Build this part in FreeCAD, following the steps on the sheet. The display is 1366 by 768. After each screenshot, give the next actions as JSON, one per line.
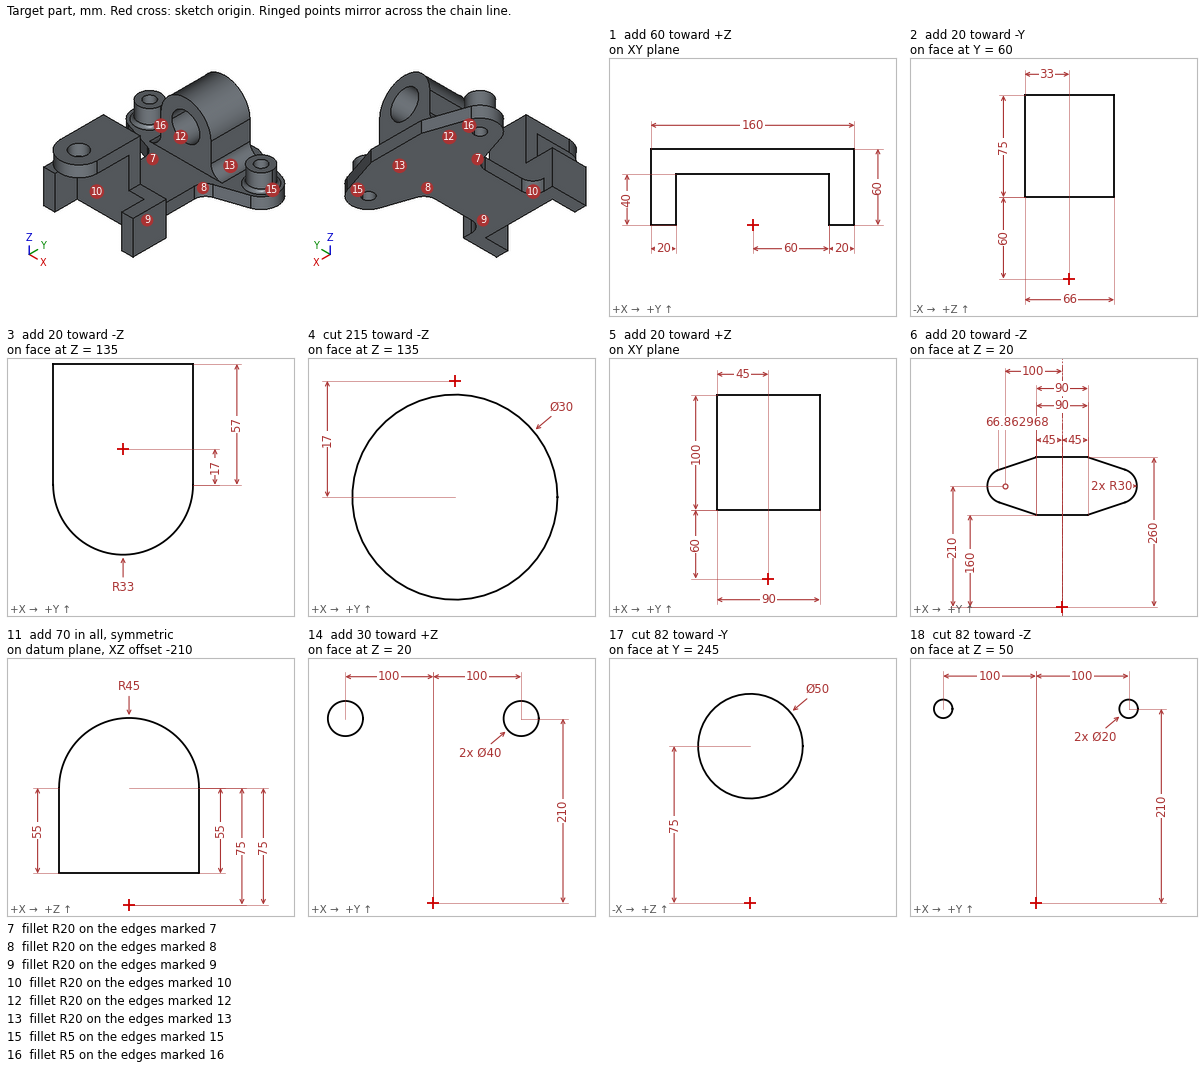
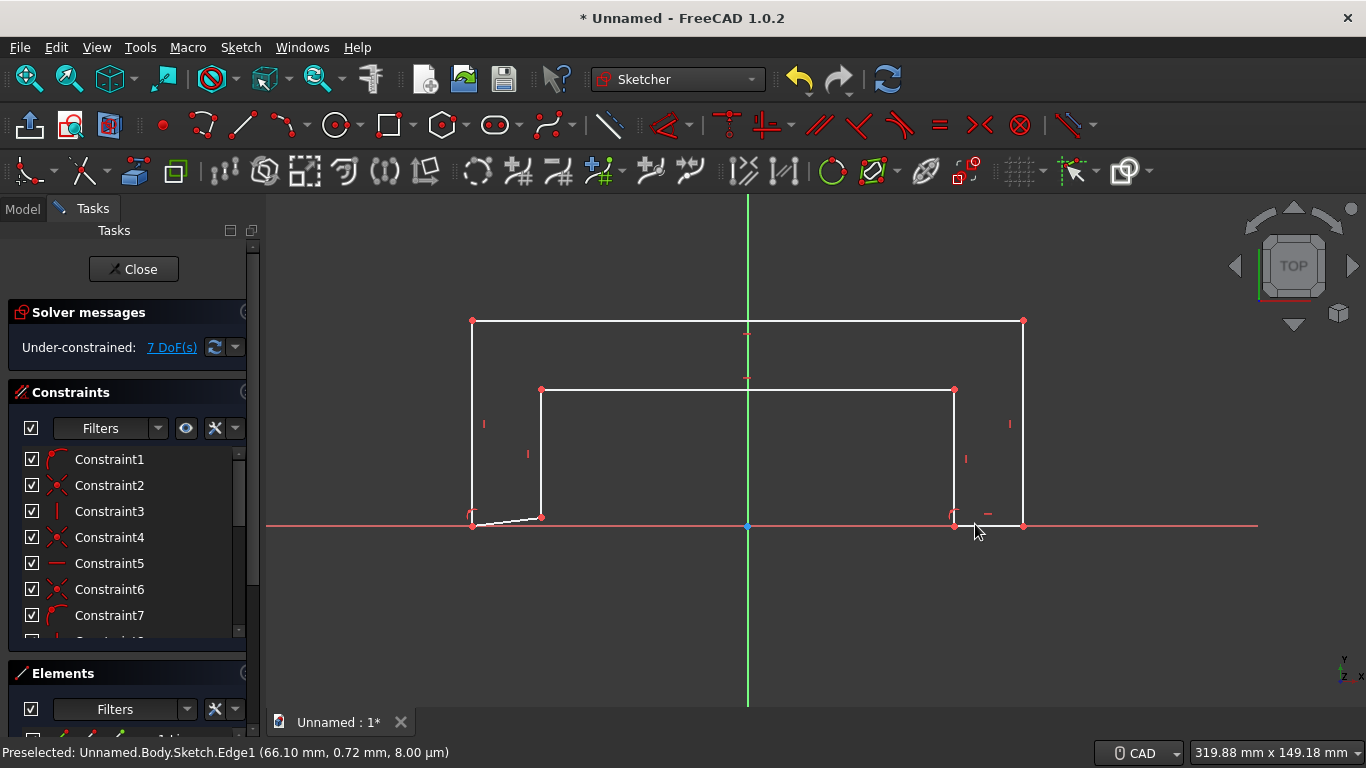
{"action": "left_click", "coordinate": [493, 524]}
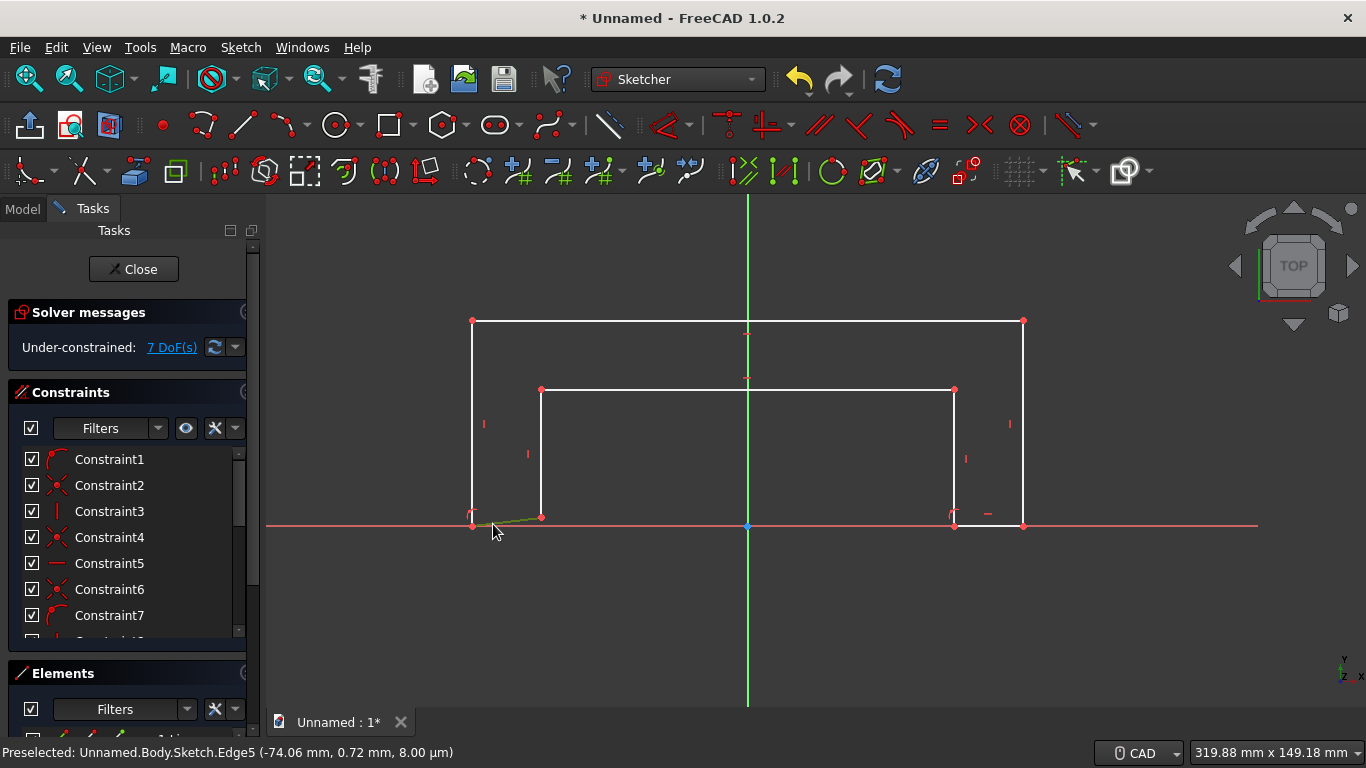
{"action": "left_click", "coordinate": [794, 126]}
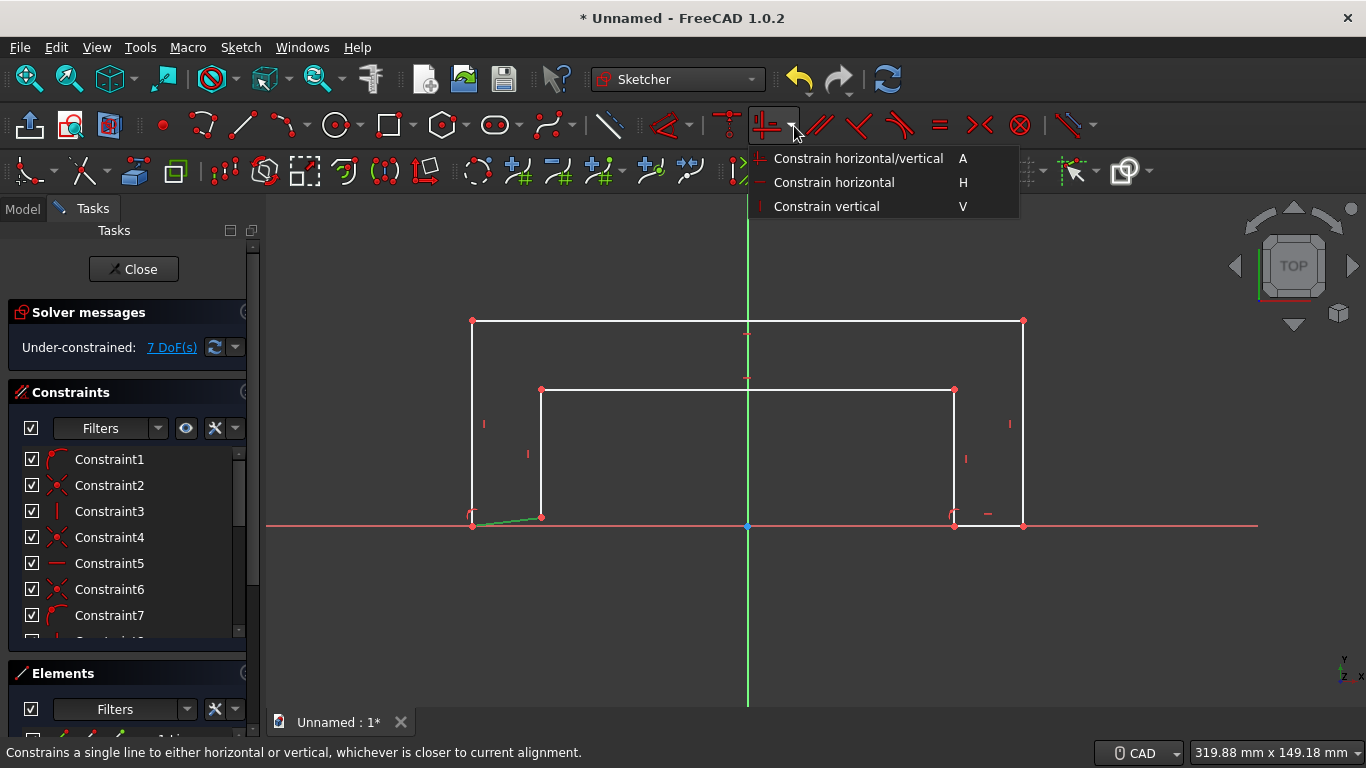
{"action": "left_click", "coordinate": [884, 182]}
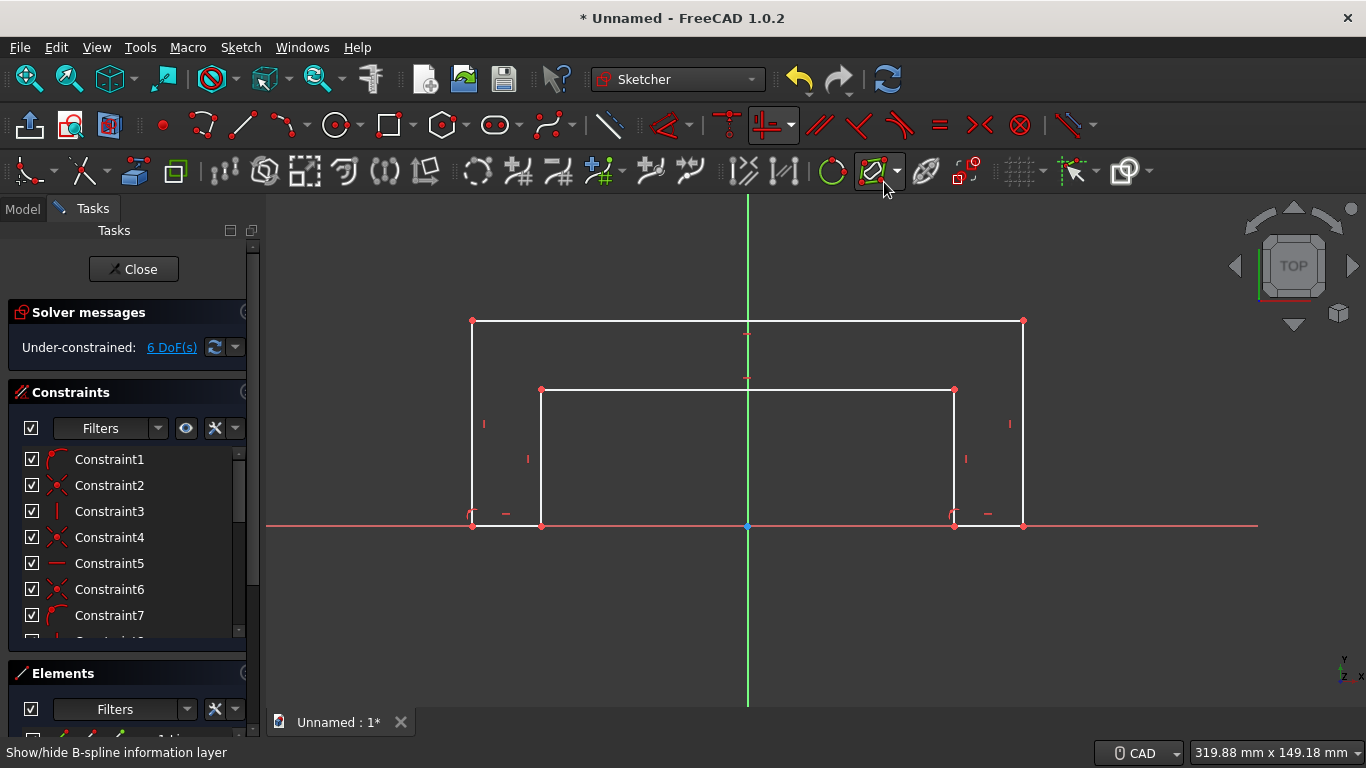
{"action": "left_click", "coordinate": [664, 126]}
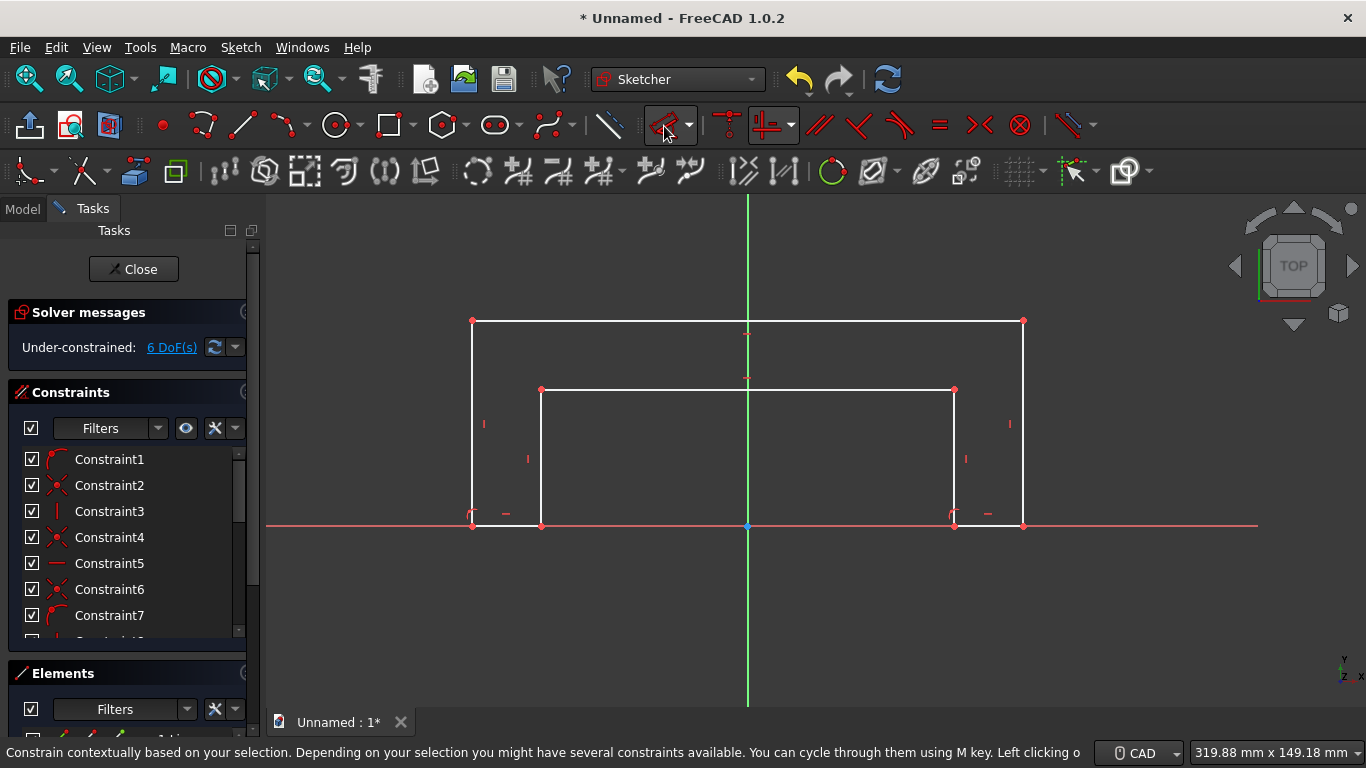
{"action": "left_click", "coordinate": [975, 526]}
{"action": "left_click", "coordinate": [989, 560]}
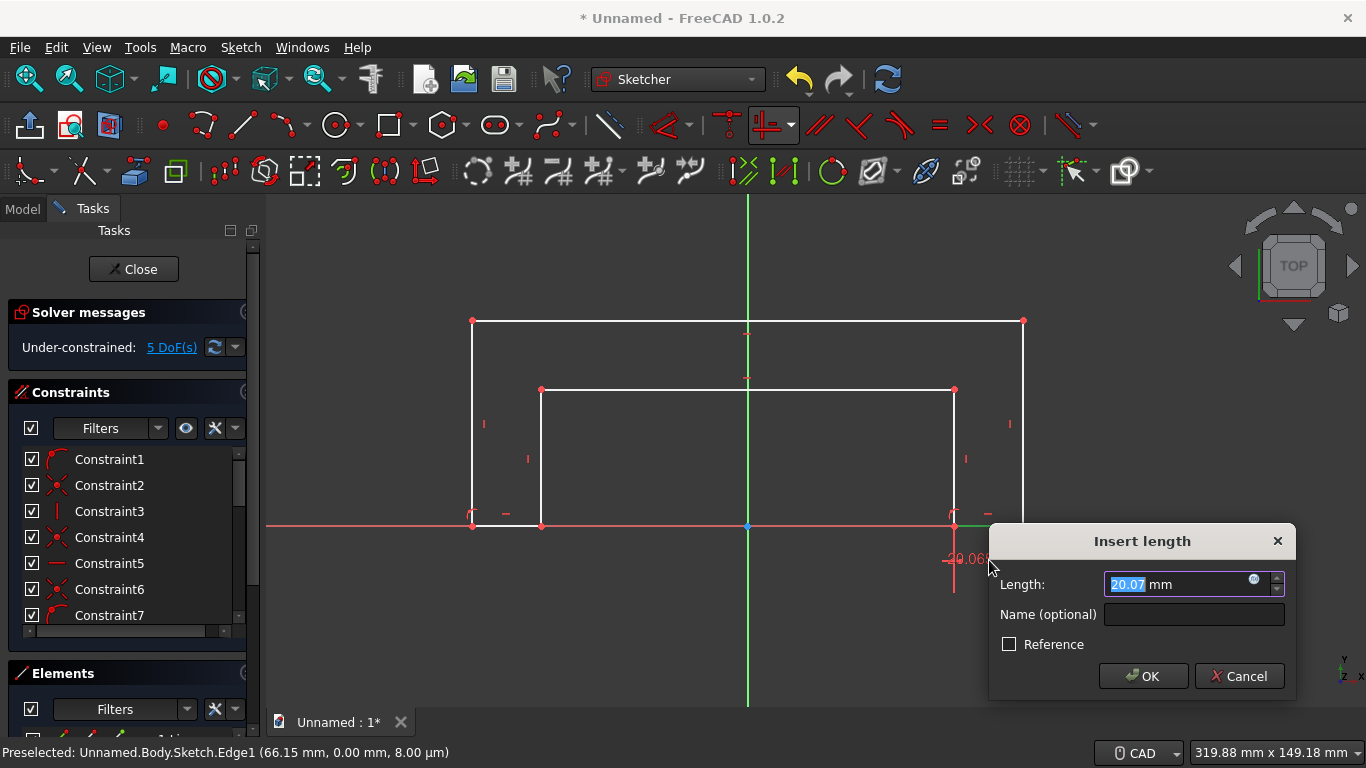
{"action": "type", "text": "20"}
{"action": "key", "text": "Return"}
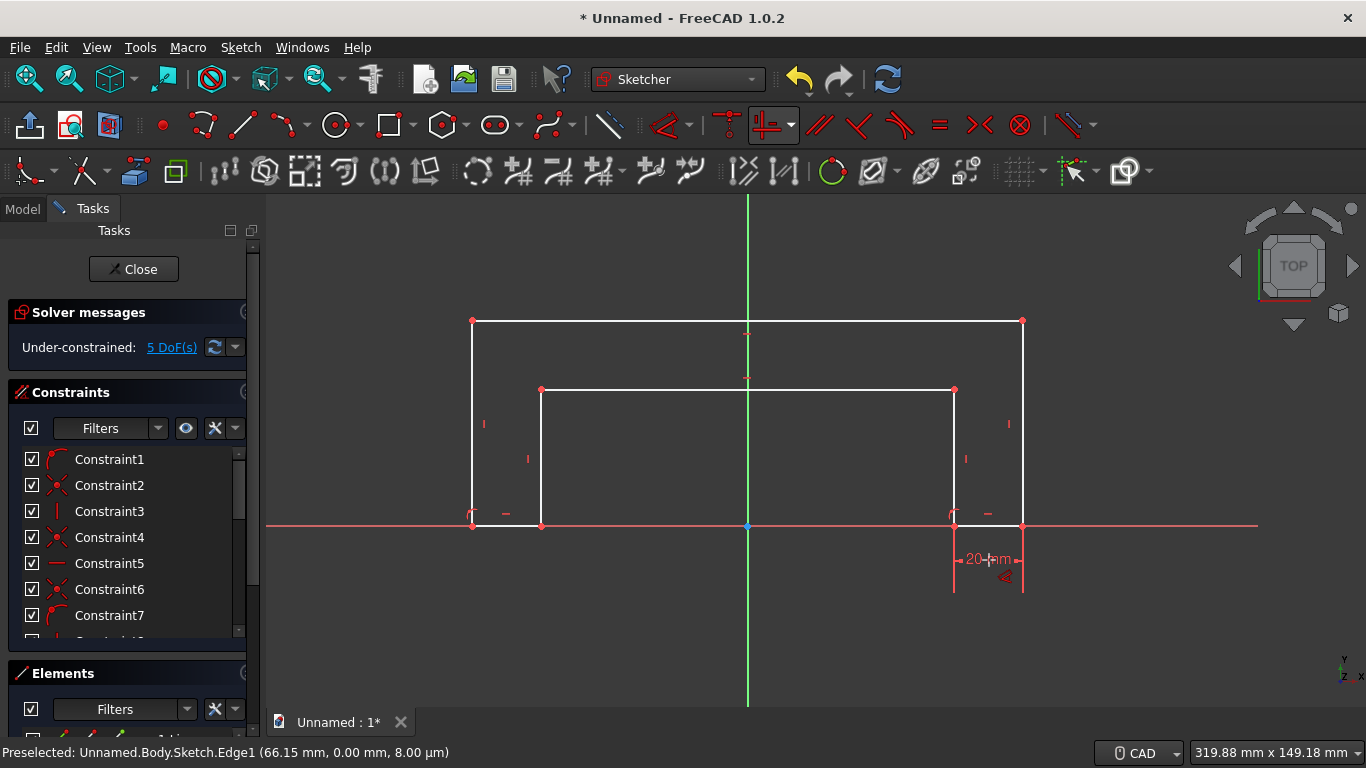
{"action": "left_click", "coordinate": [1023, 465]}
{"action": "left_click", "coordinate": [1057, 424]}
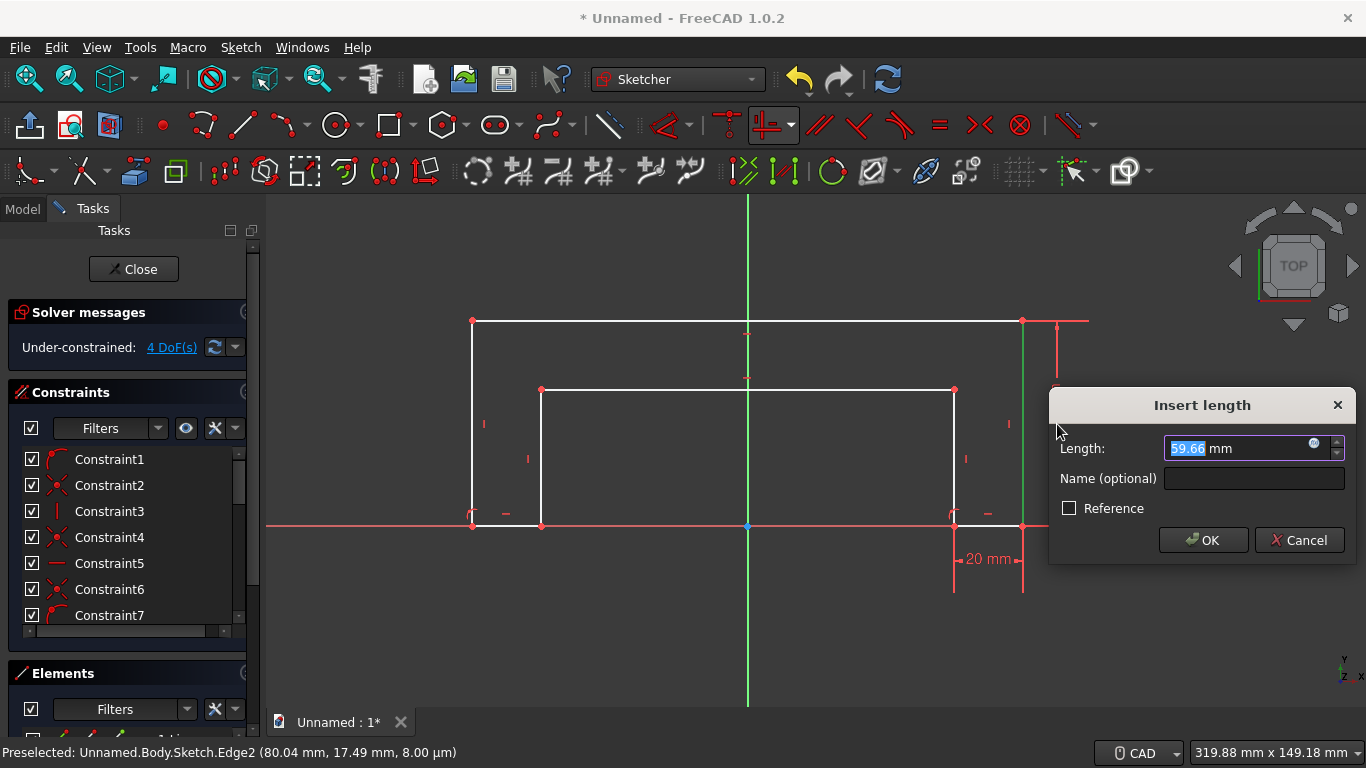
{"action": "type", "text": "60"}
{"action": "key", "text": "Return"}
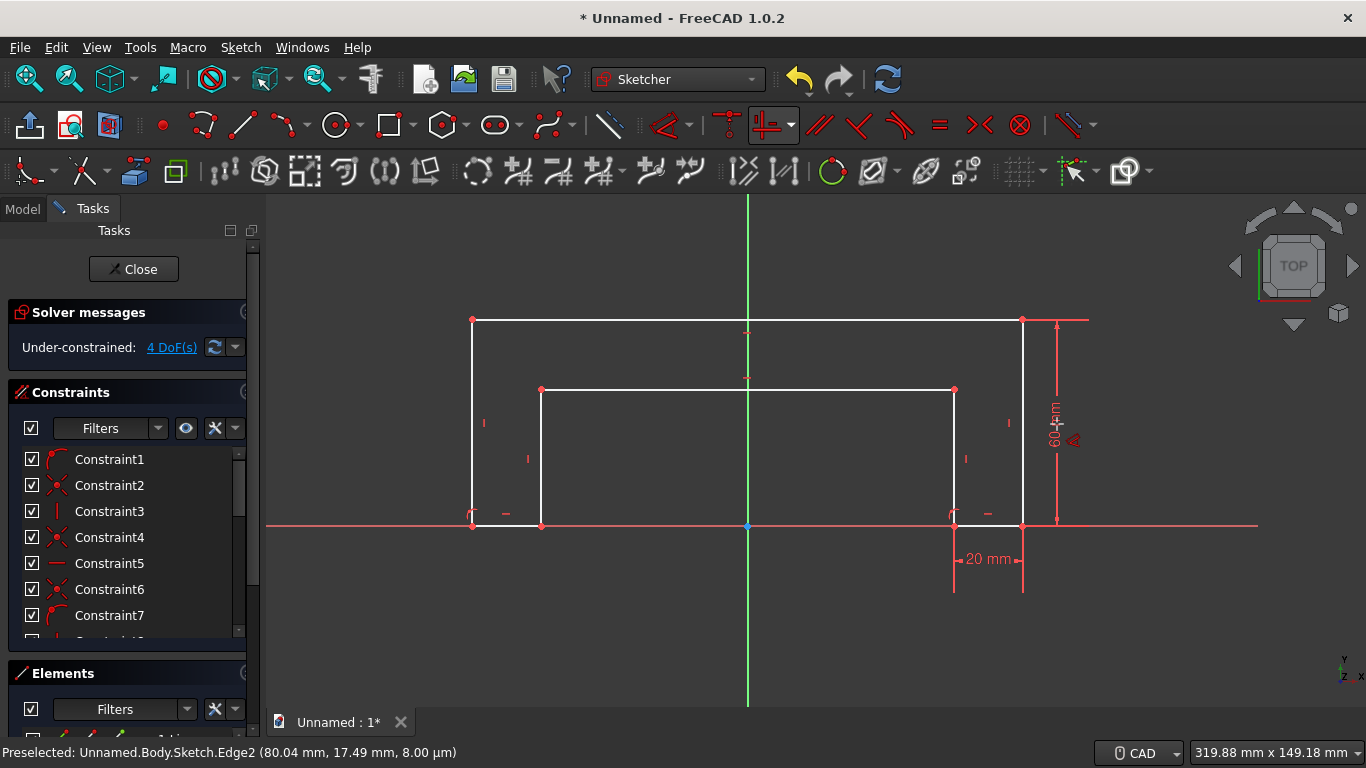
{"action": "left_click", "coordinate": [493, 526]}
{"action": "left_click", "coordinate": [507, 560]}